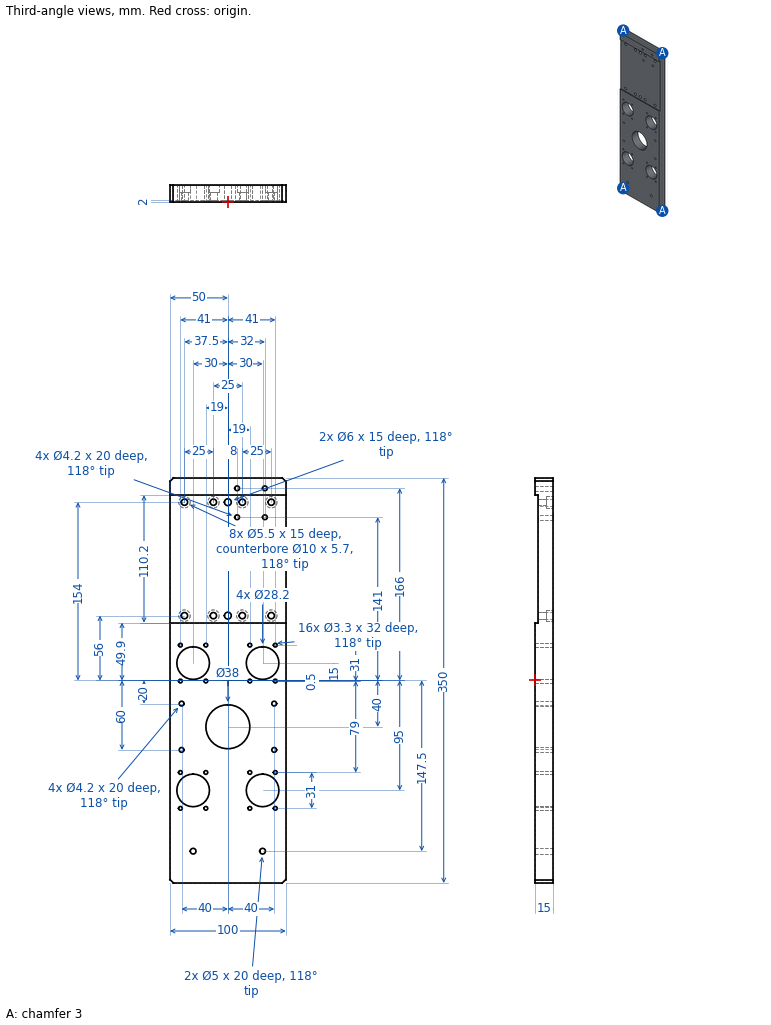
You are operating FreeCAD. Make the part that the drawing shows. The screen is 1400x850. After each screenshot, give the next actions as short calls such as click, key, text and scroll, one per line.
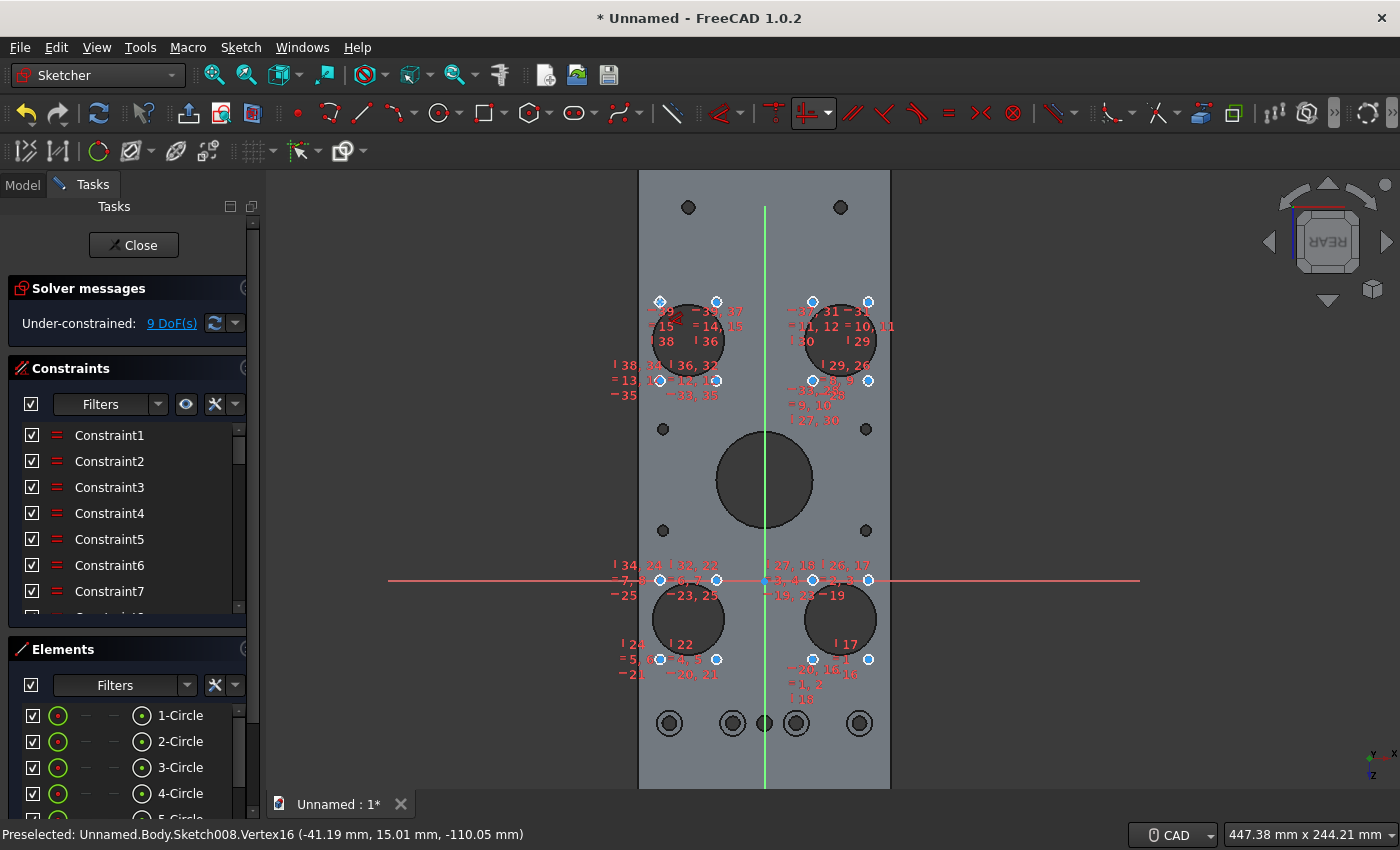
scroll(872, 663, up, 8)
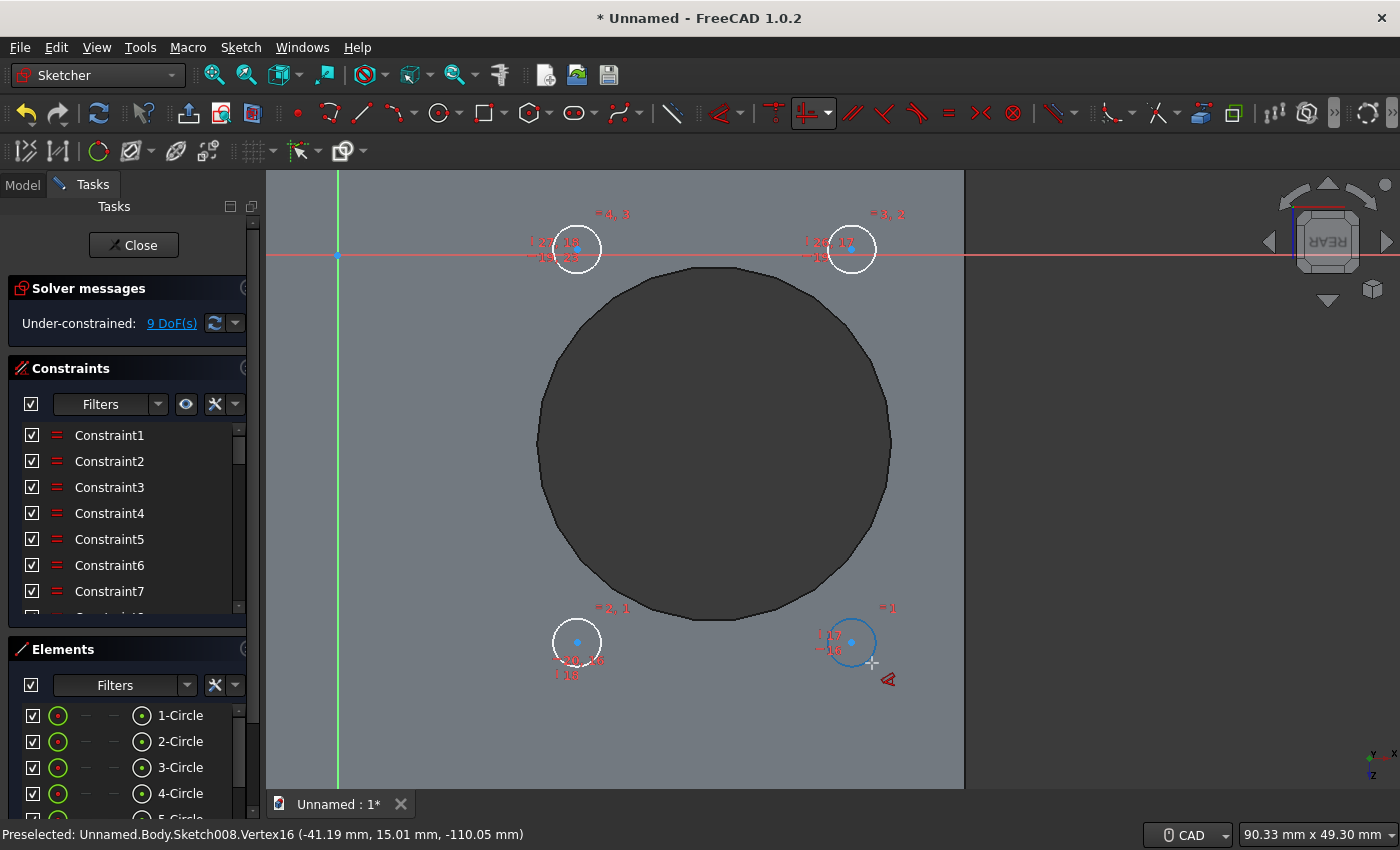
click(869, 660)
click(892, 683)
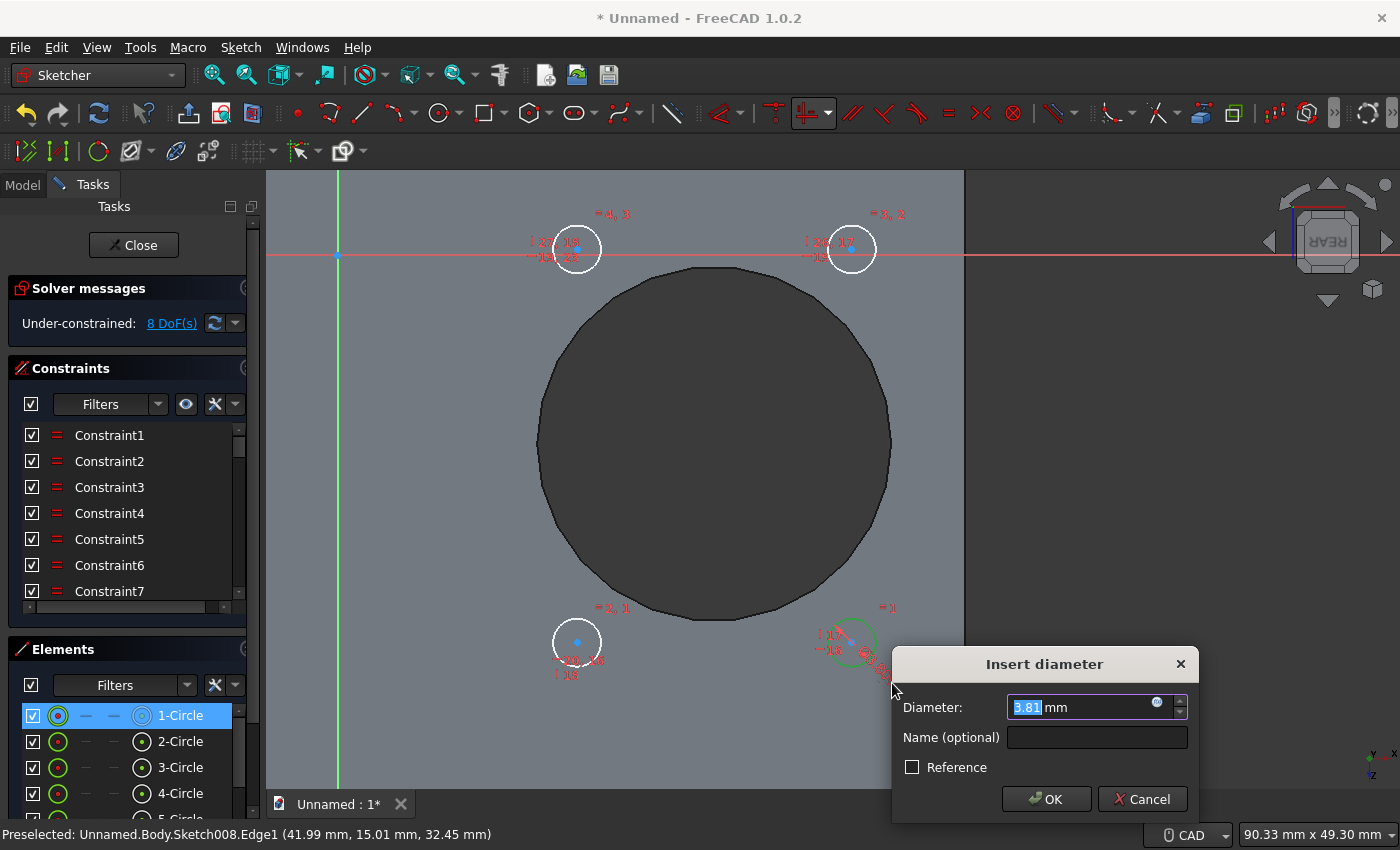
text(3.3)
key(Return)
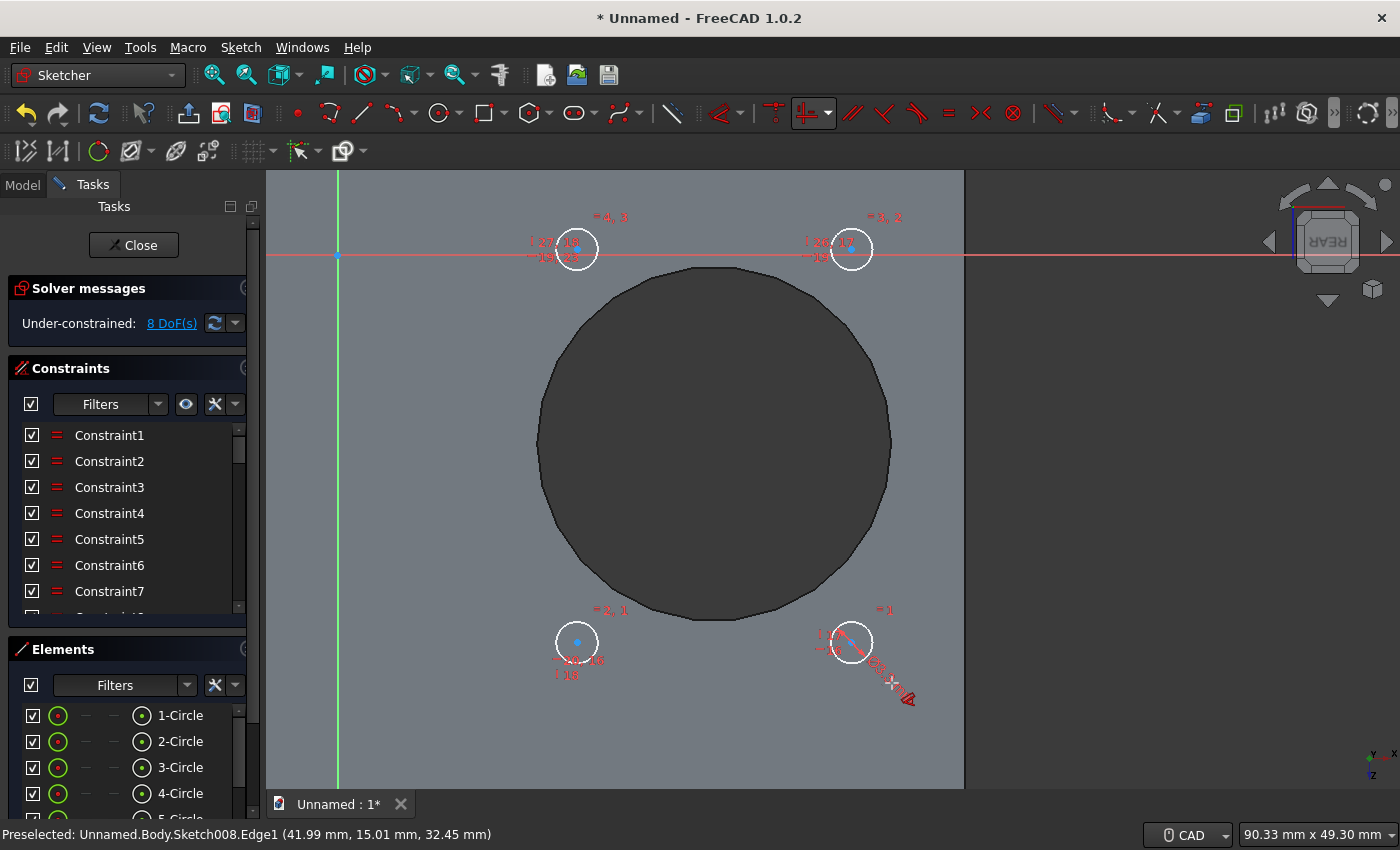
scroll(873, 663, down, 8)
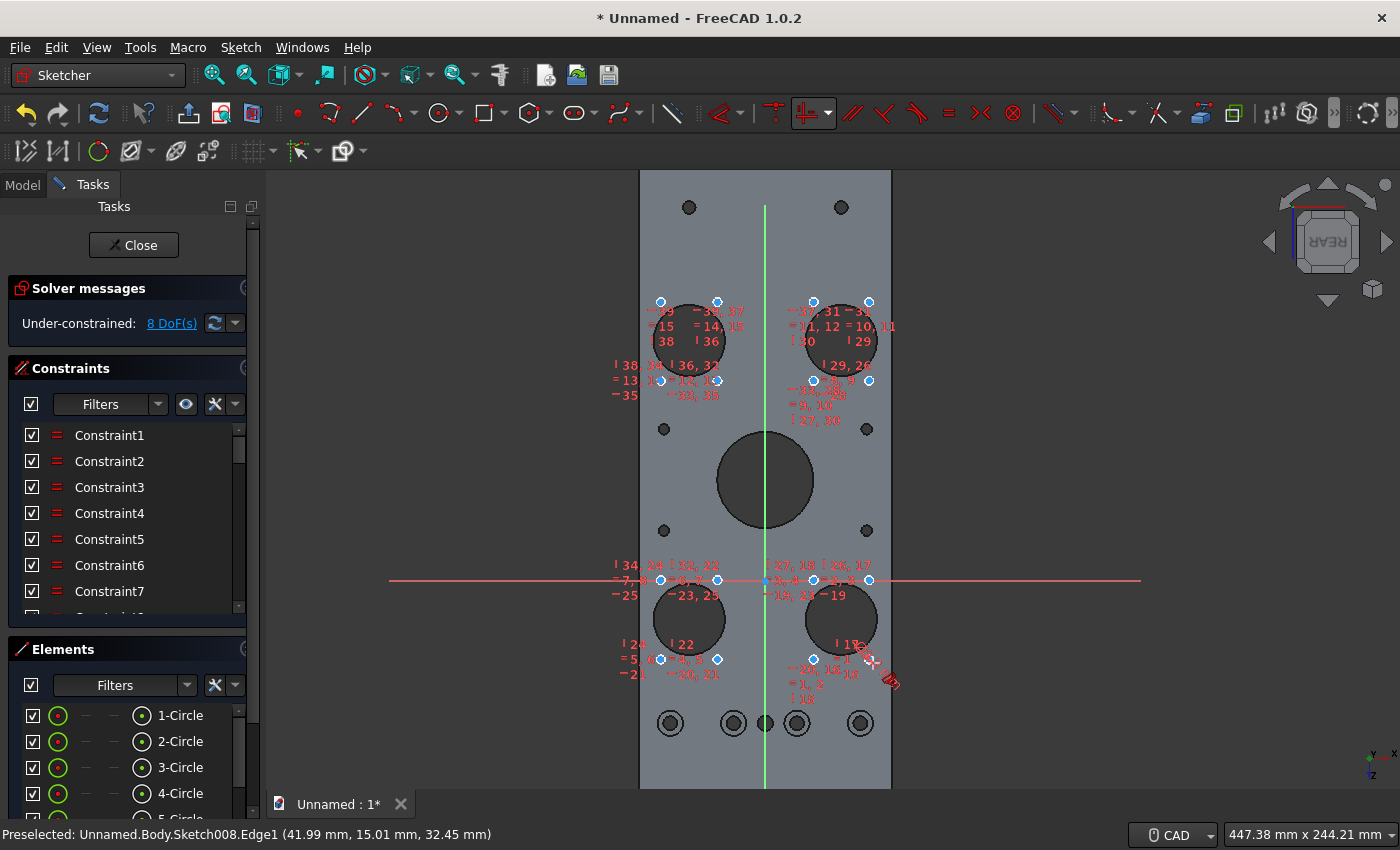
click(869, 660)
click(817, 694)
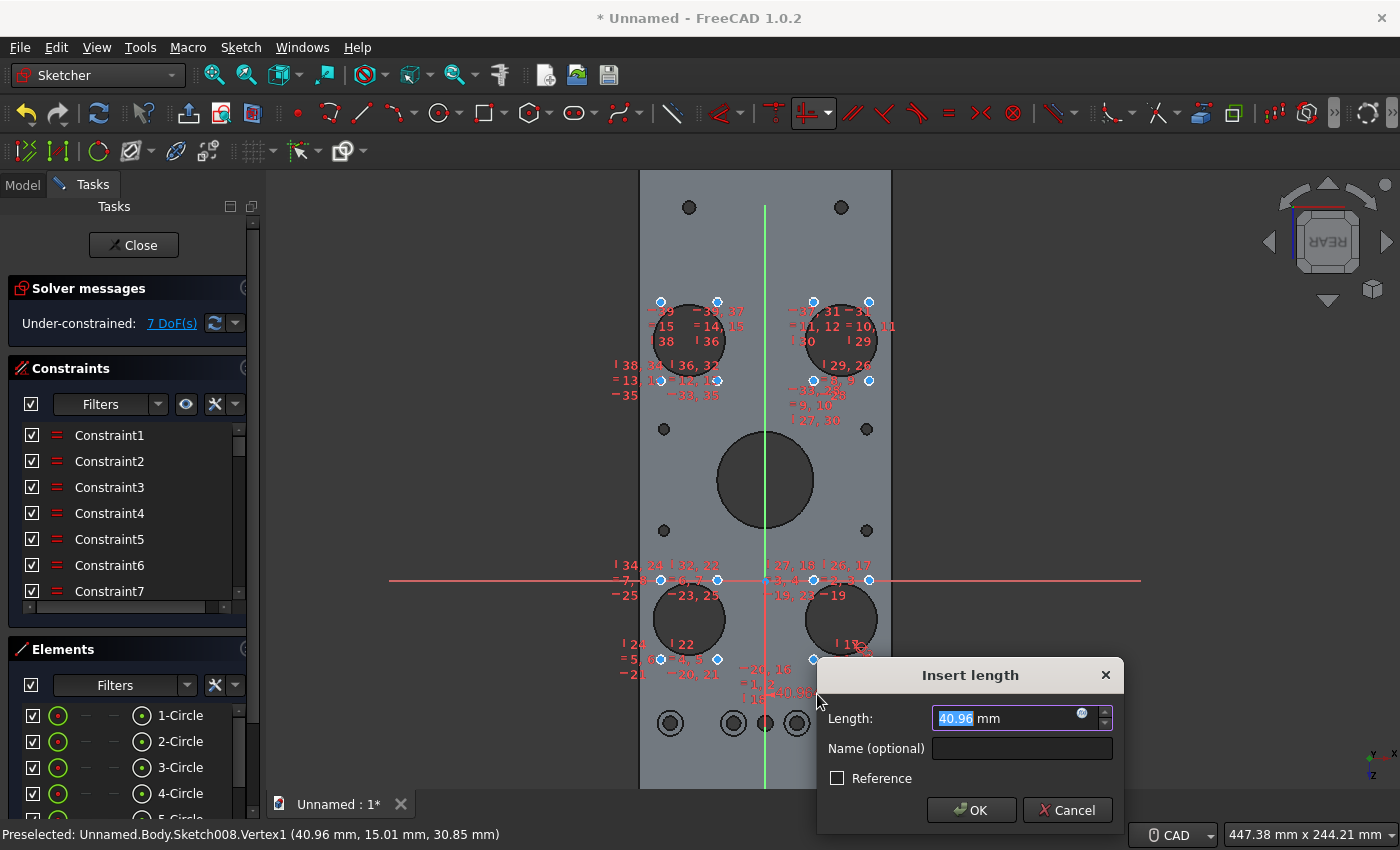
text(41)
key(Return)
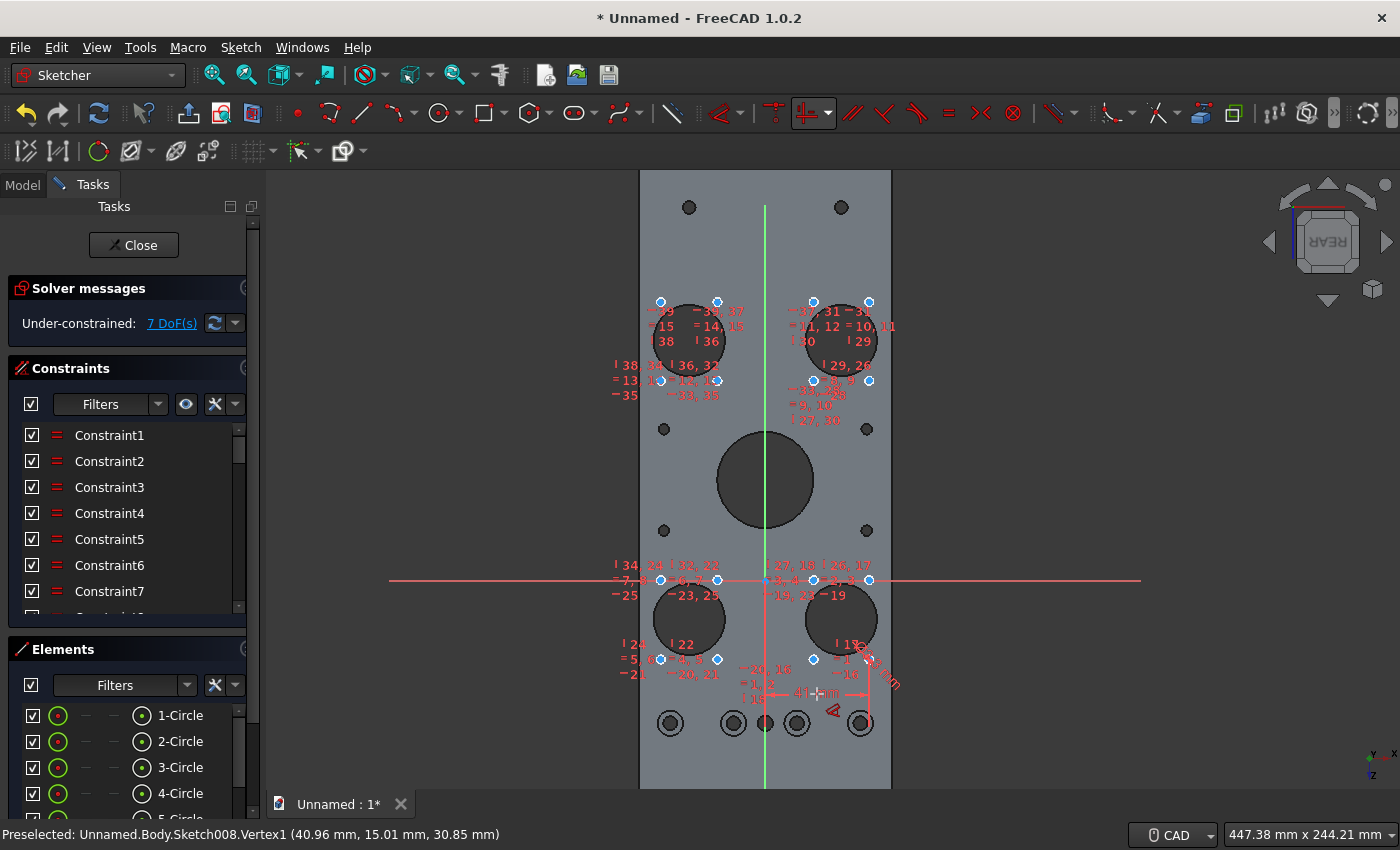
click(814, 660)
click(789, 547)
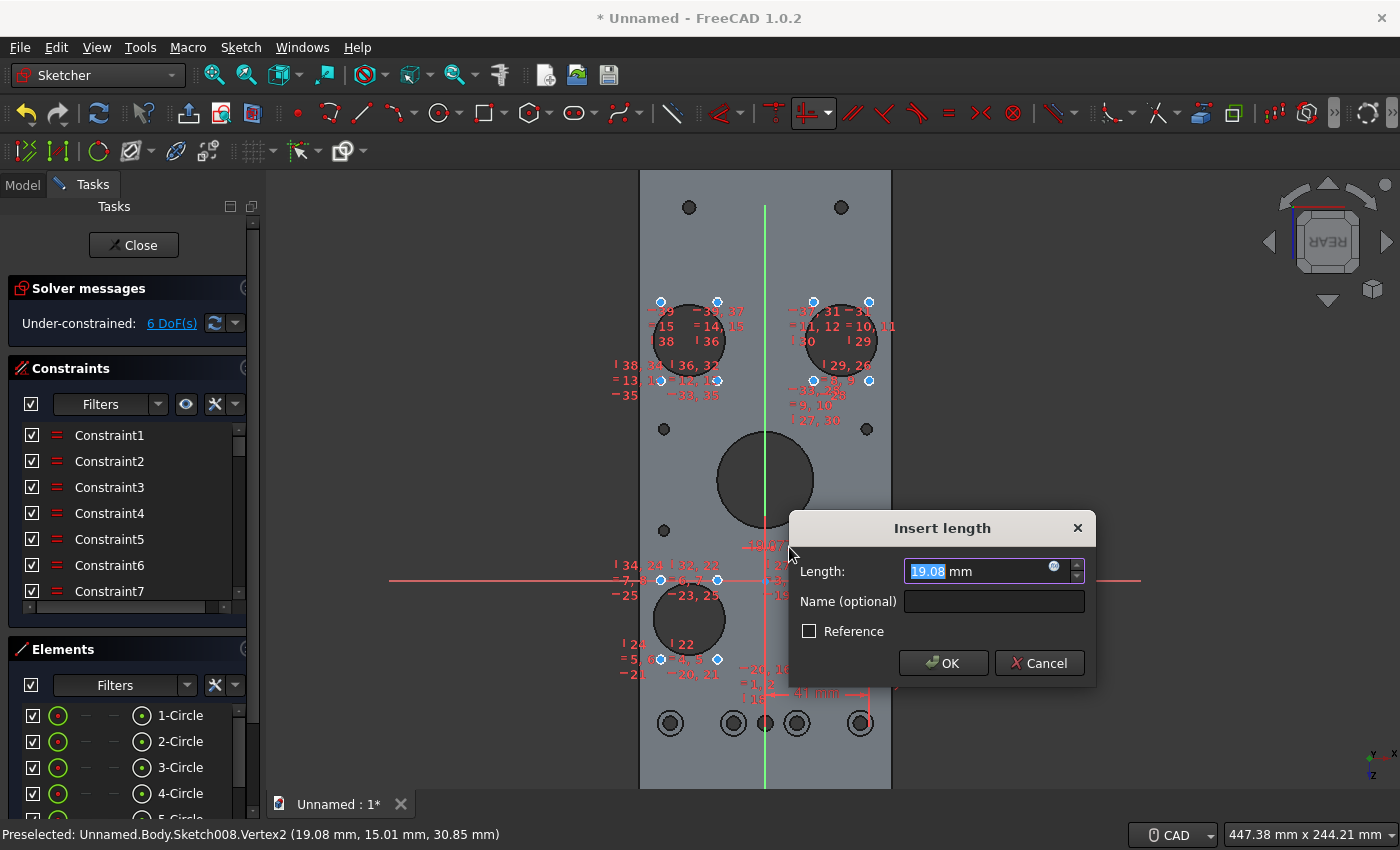
text(19)
key(Return)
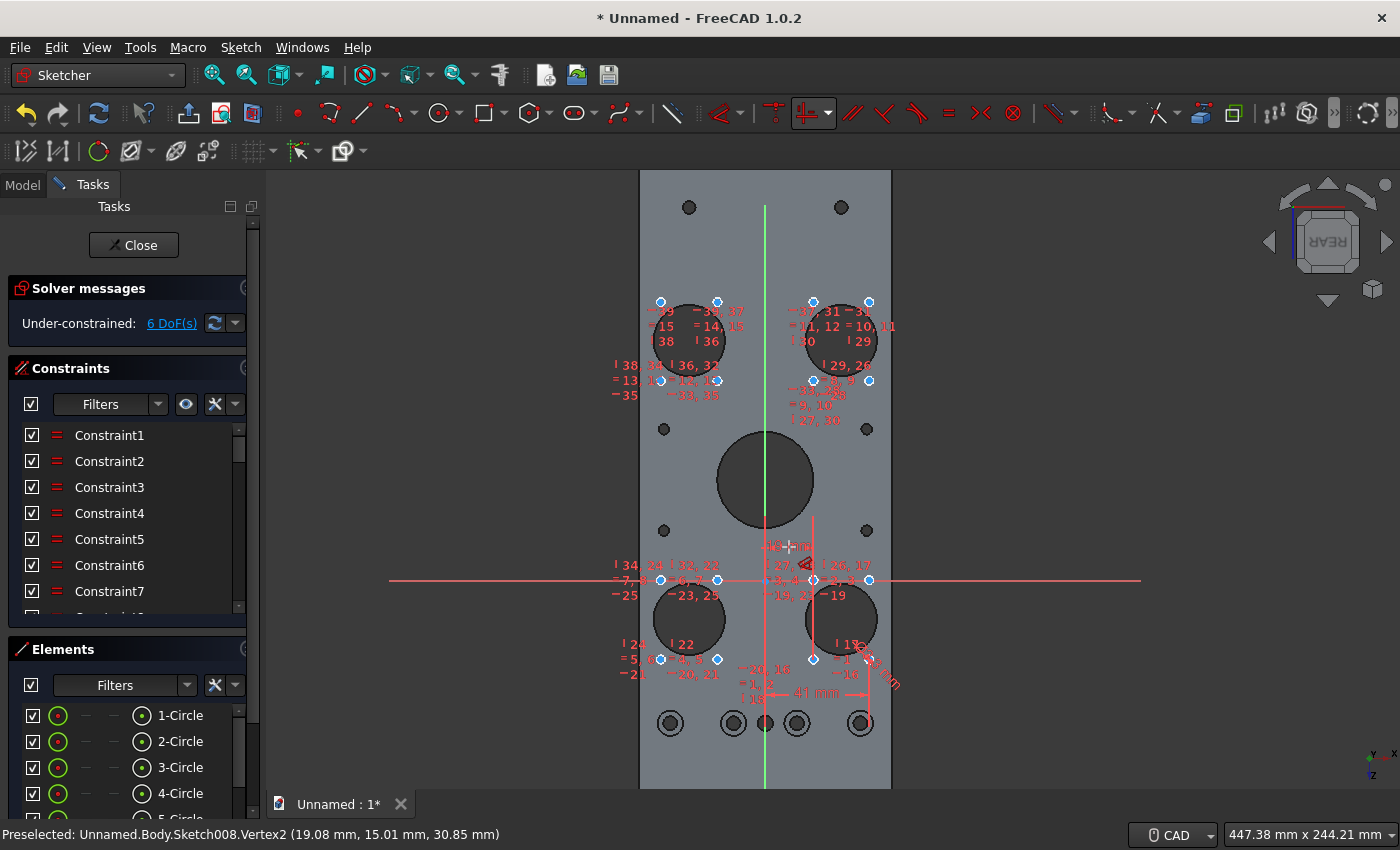
click(717, 660)
click(741, 694)